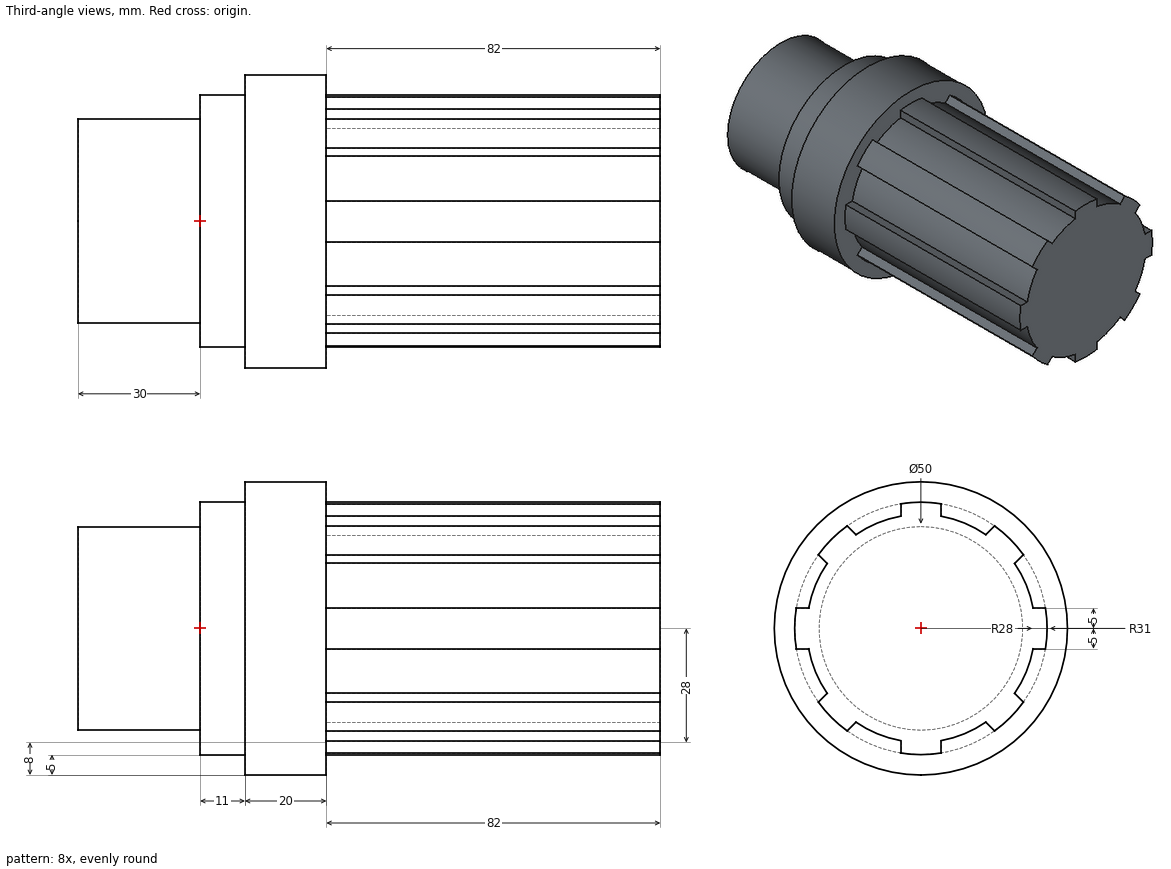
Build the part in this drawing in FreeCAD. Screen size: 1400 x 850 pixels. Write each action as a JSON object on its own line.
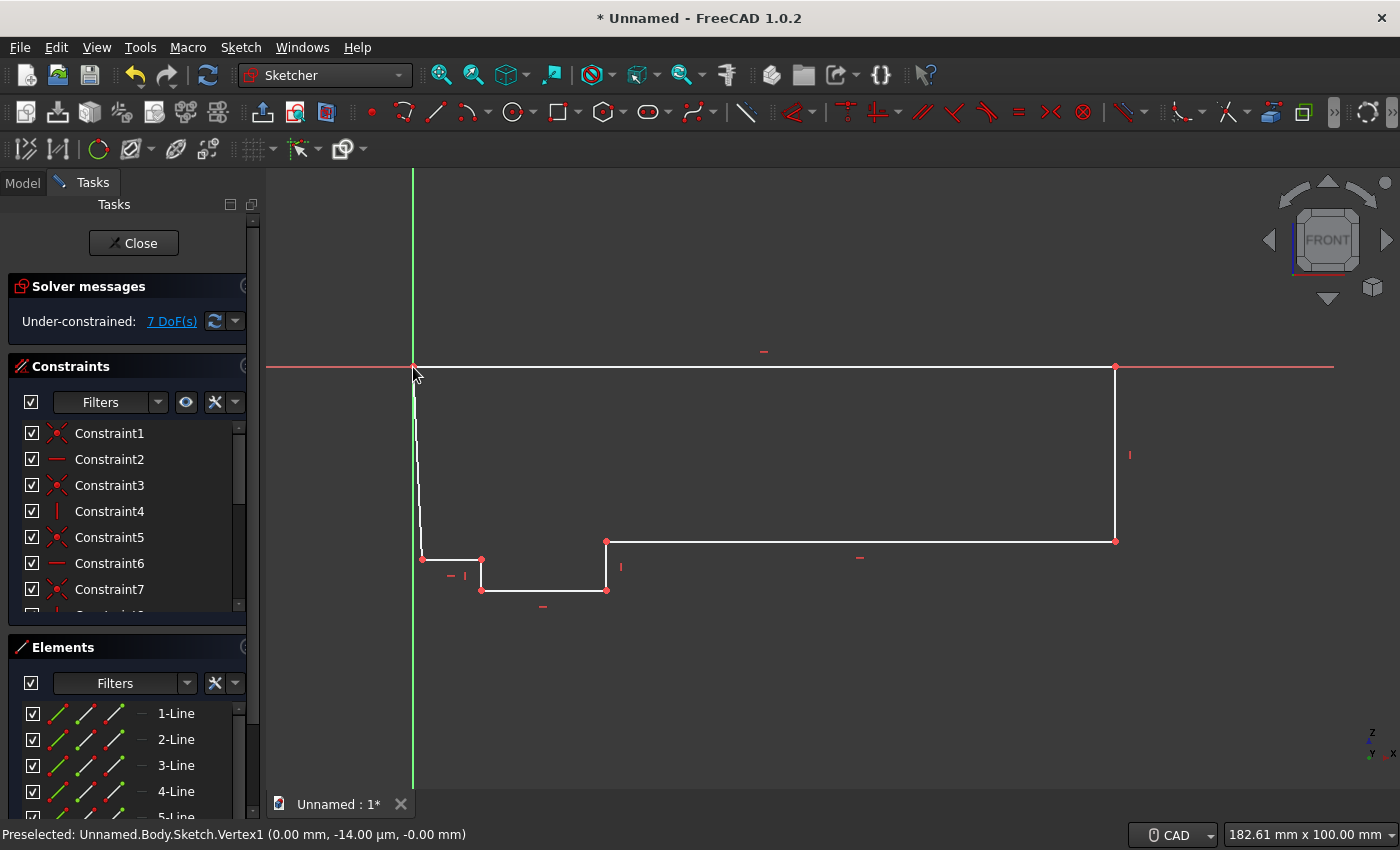
{"action": "left_click", "coordinate": [416, 425]}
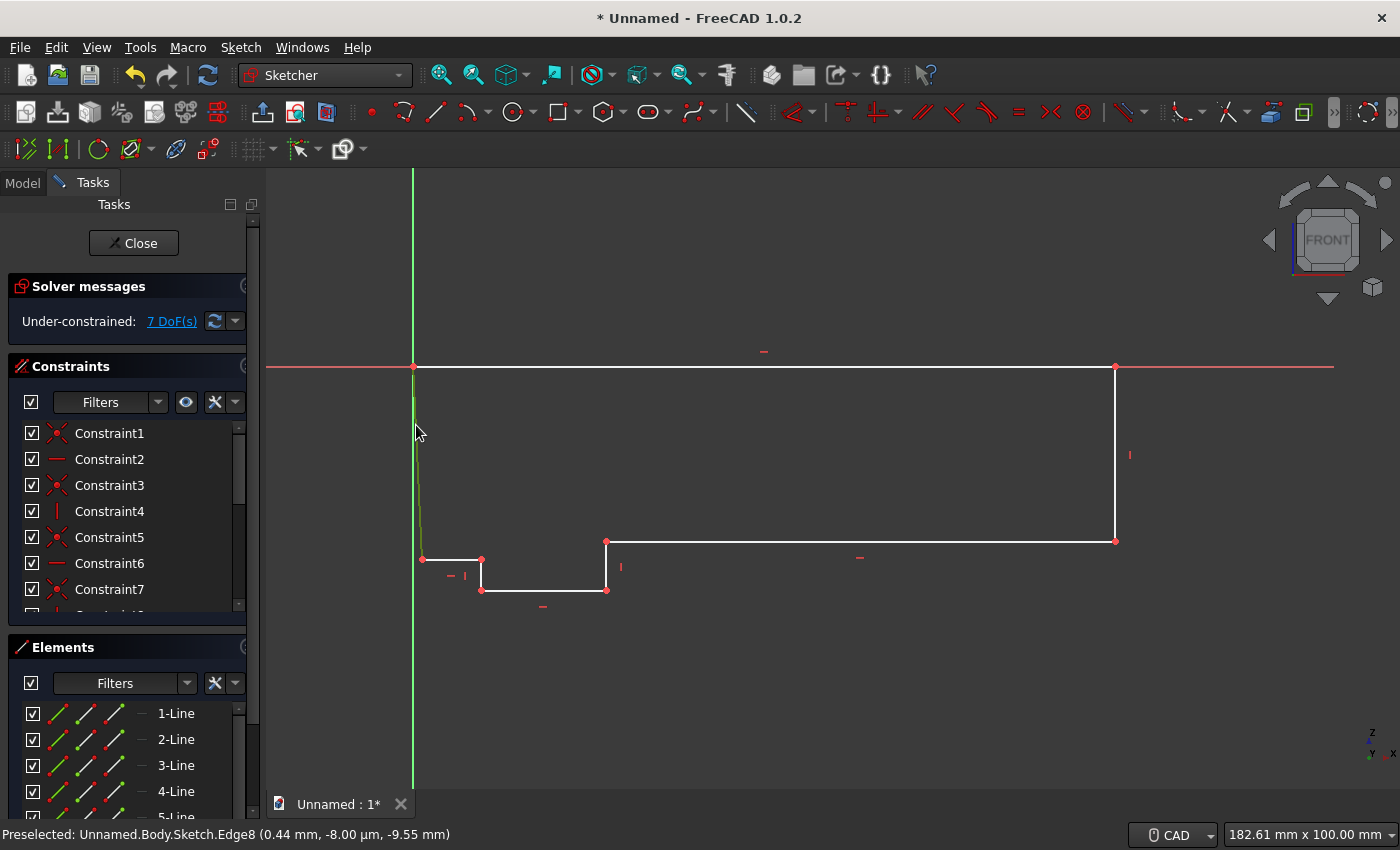
{"action": "left_click", "coordinate": [900, 112]}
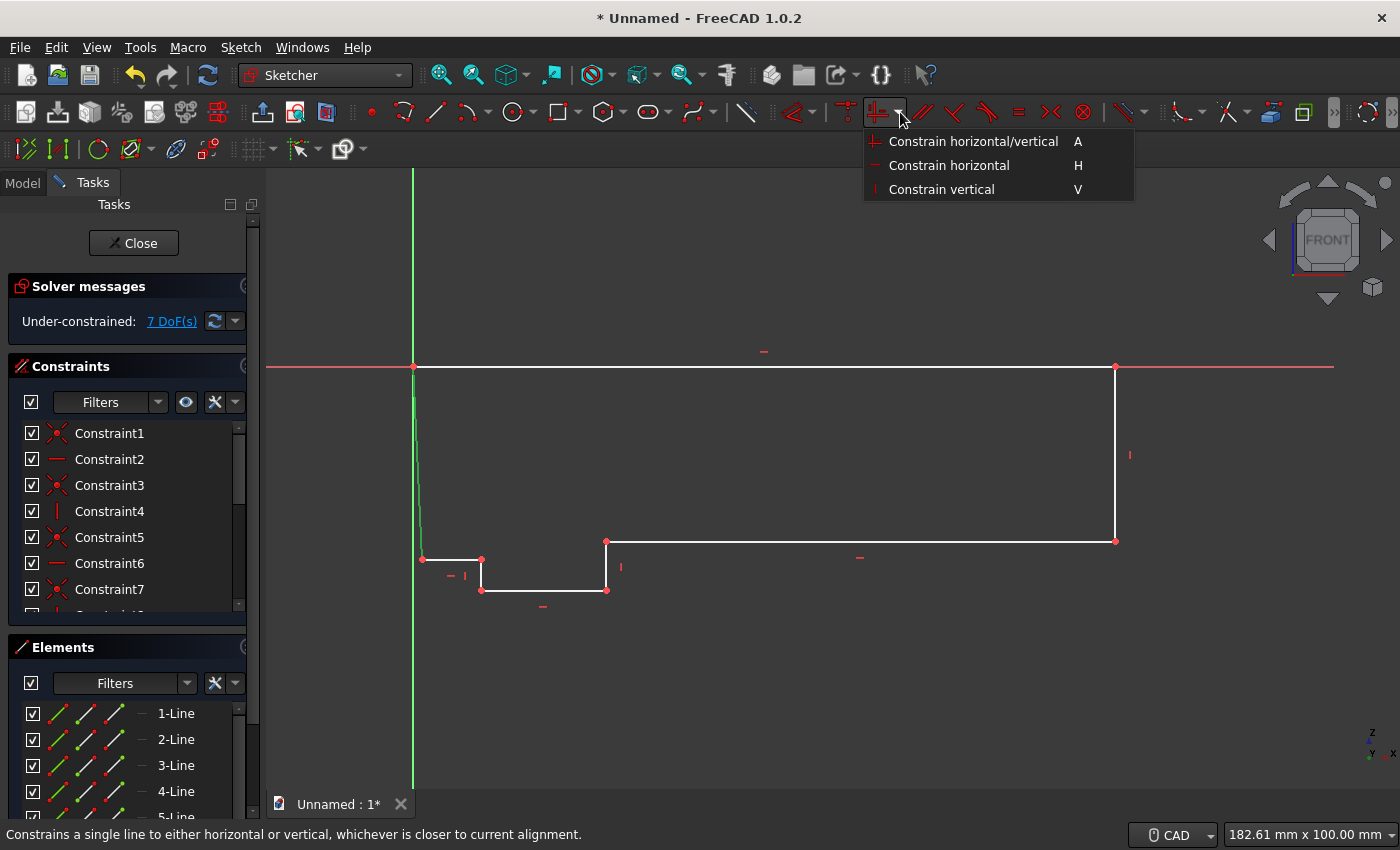
{"action": "left_click", "coordinate": [999, 189]}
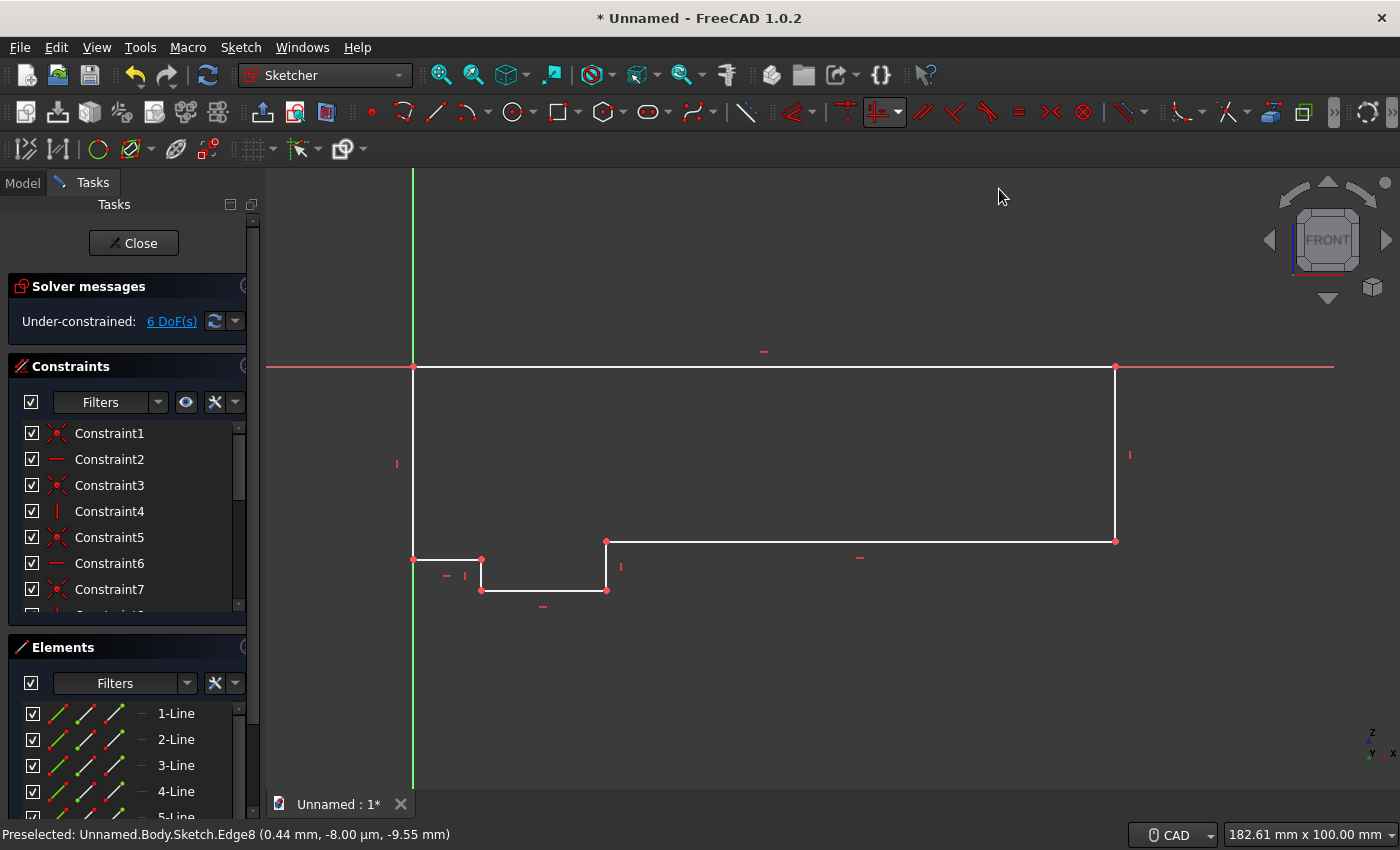
{"action": "left_click", "coordinate": [606, 557]}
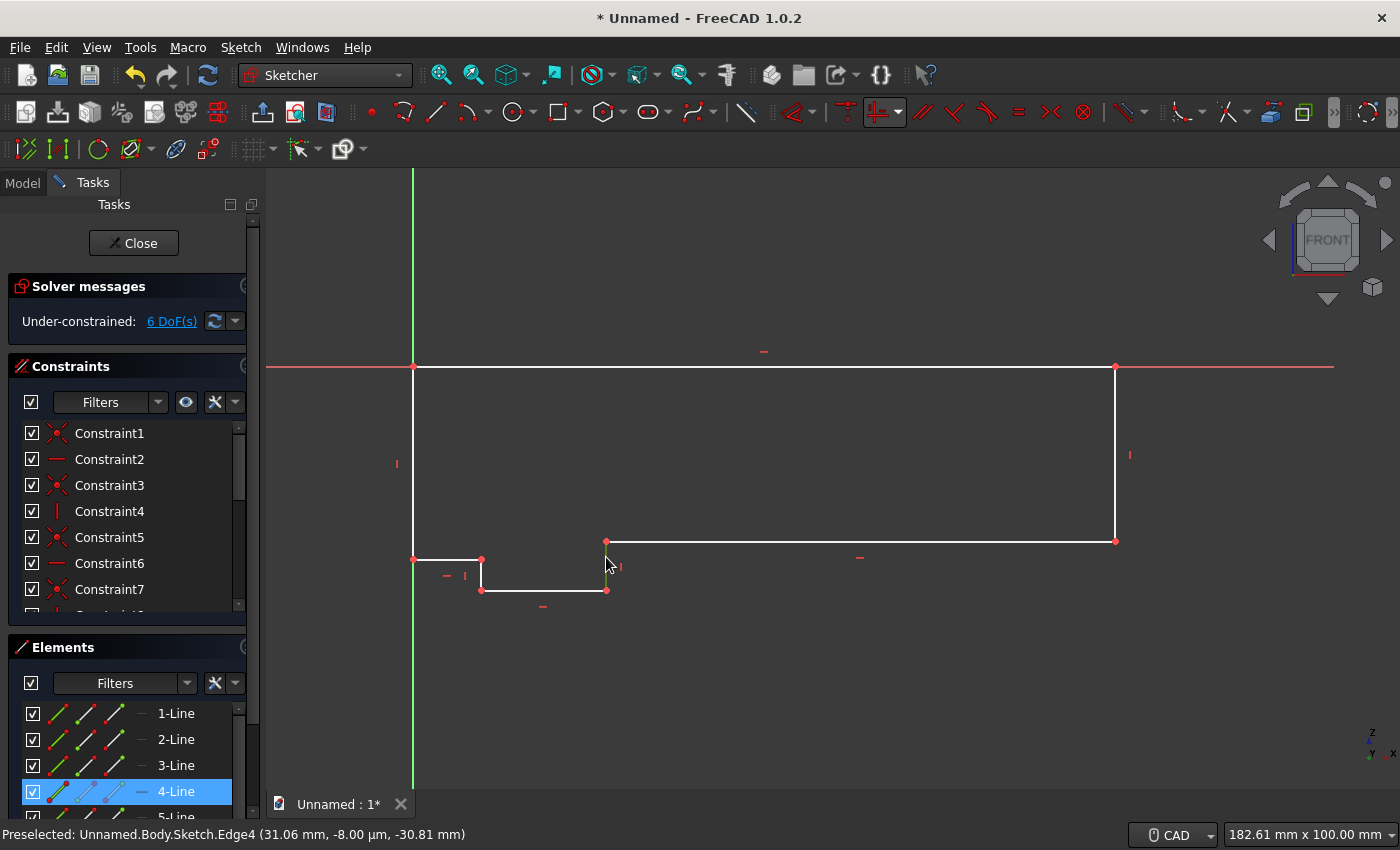
{"action": "key", "text": "i"}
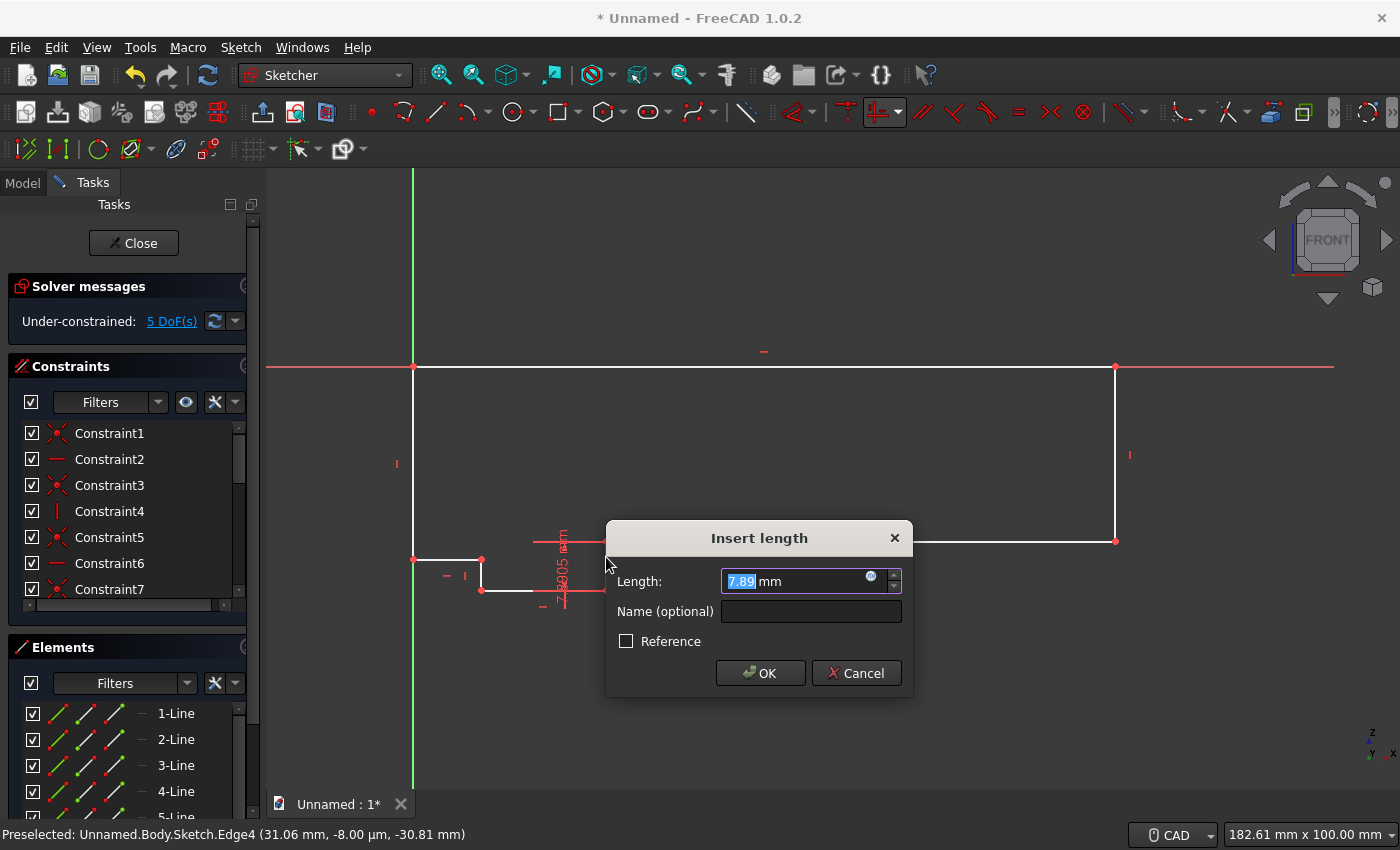
{"action": "type", "text": "8"}
{"action": "key", "text": "Return"}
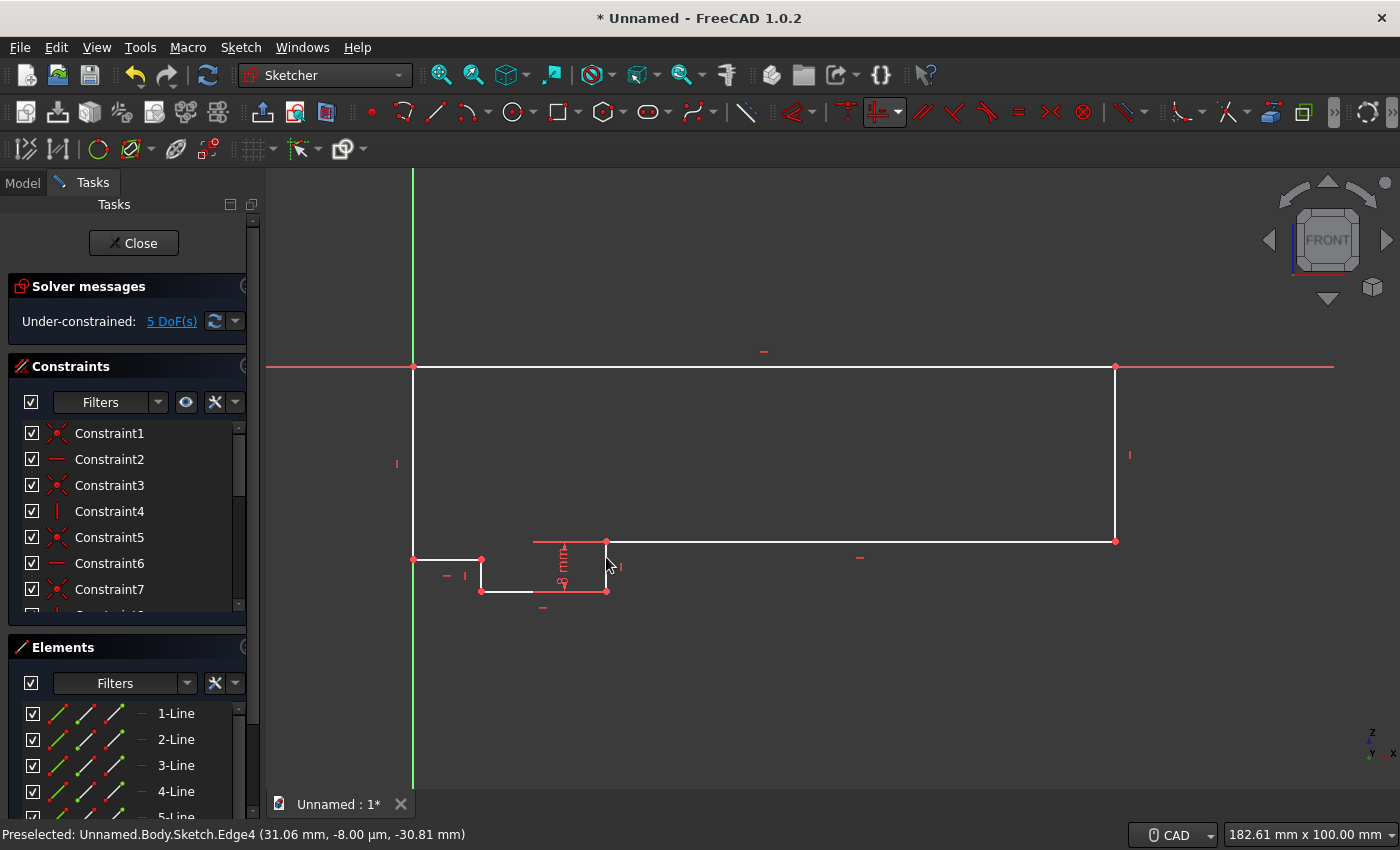
{"action": "scroll", "coordinate": [481, 582], "scroll_direction": "up", "scroll_amount": 2}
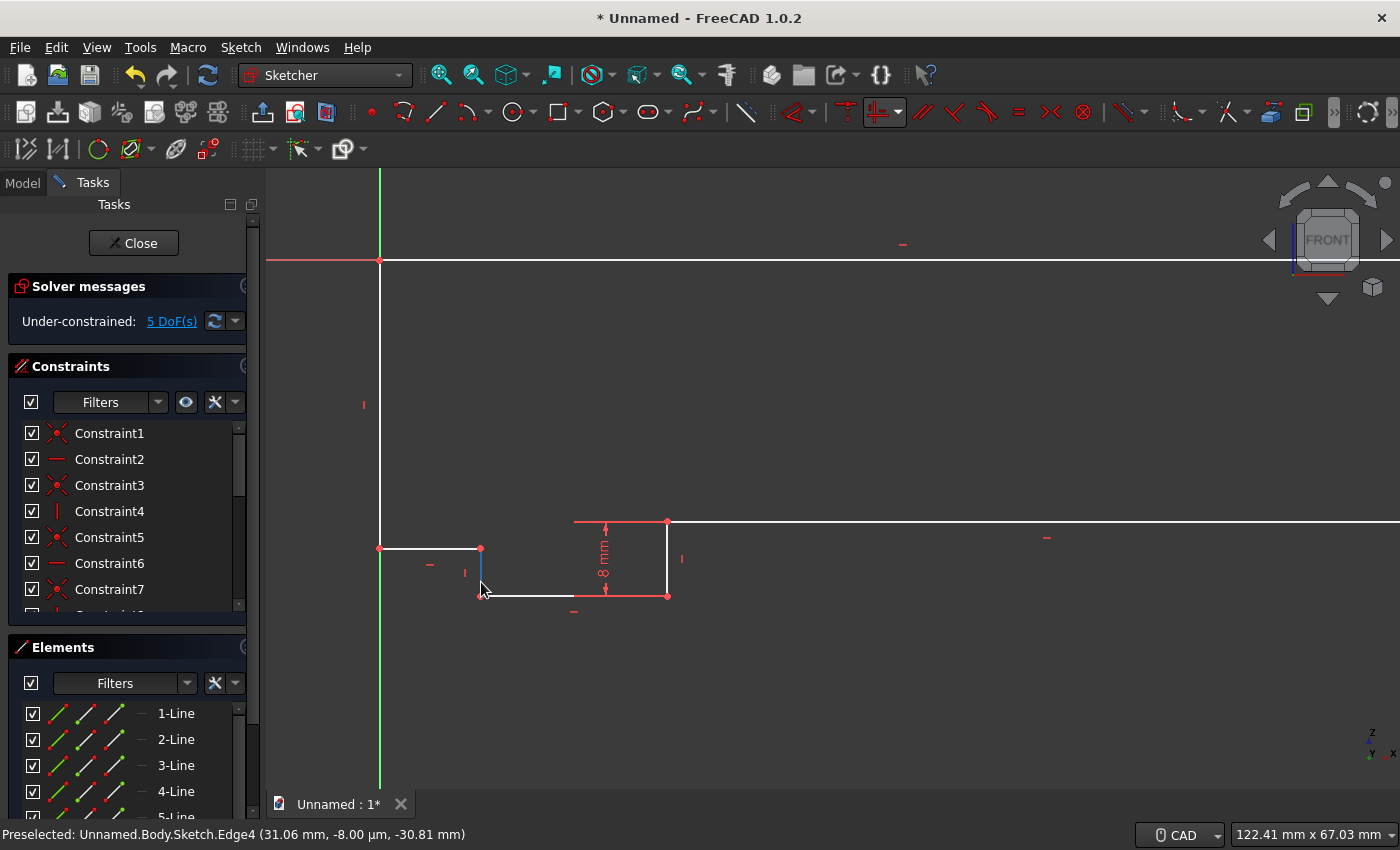
{"action": "left_click", "coordinate": [481, 582]}